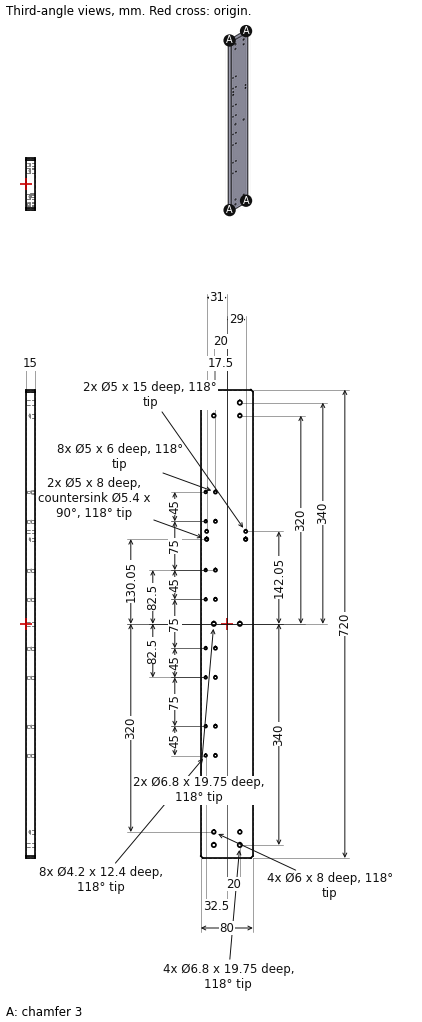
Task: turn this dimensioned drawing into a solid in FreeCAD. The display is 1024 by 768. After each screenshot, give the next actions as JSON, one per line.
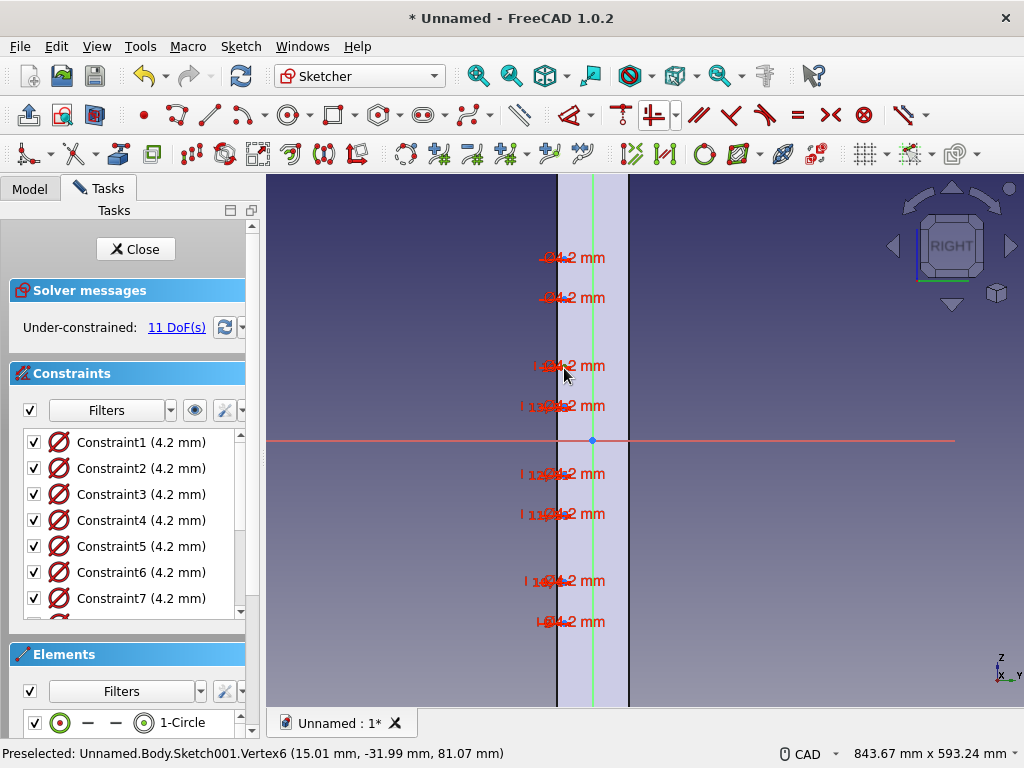
{"action": "left_click", "coordinate": [564, 300]}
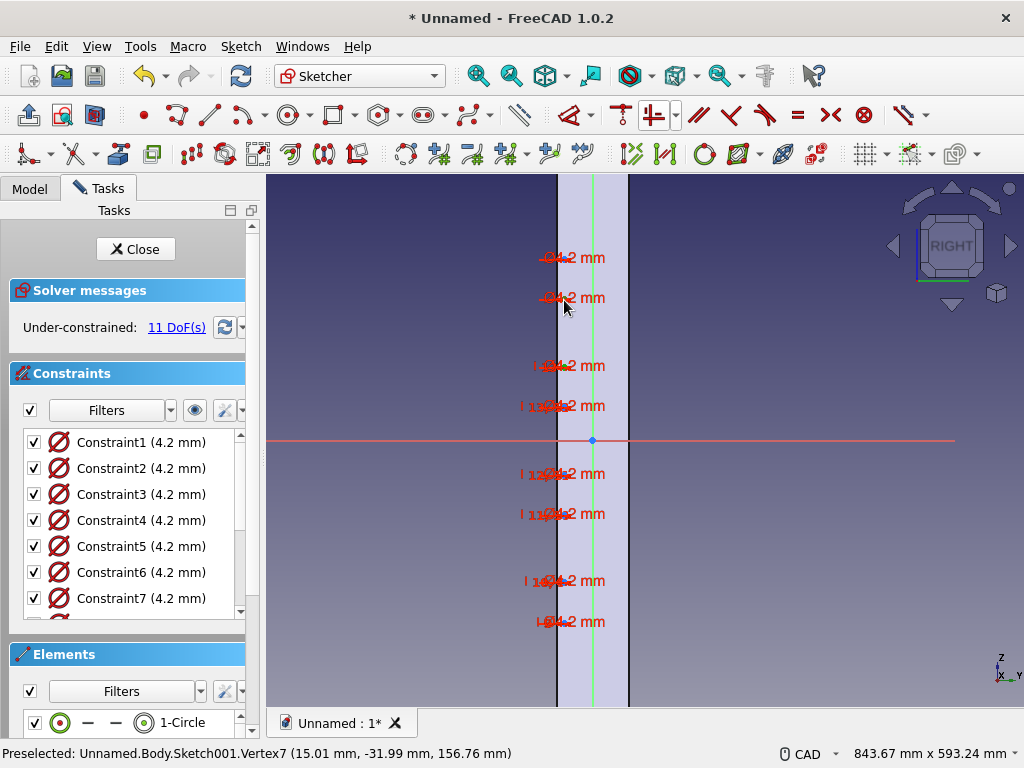
{"action": "left_click", "coordinate": [676, 116]}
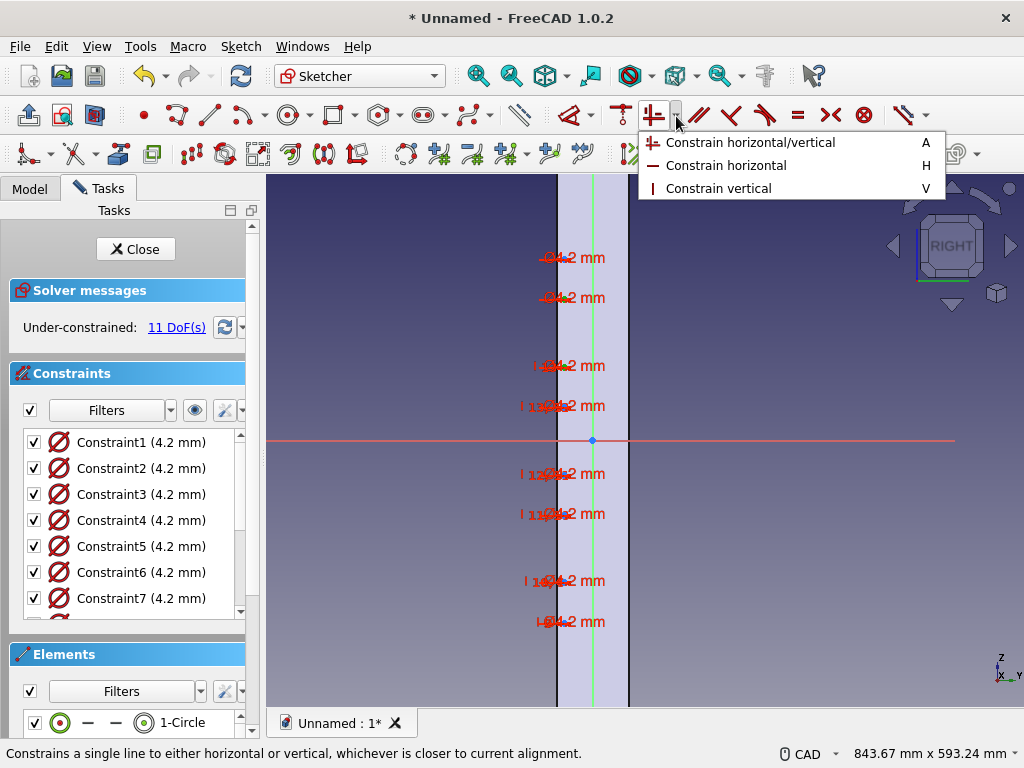
{"action": "left_click", "coordinate": [792, 188]}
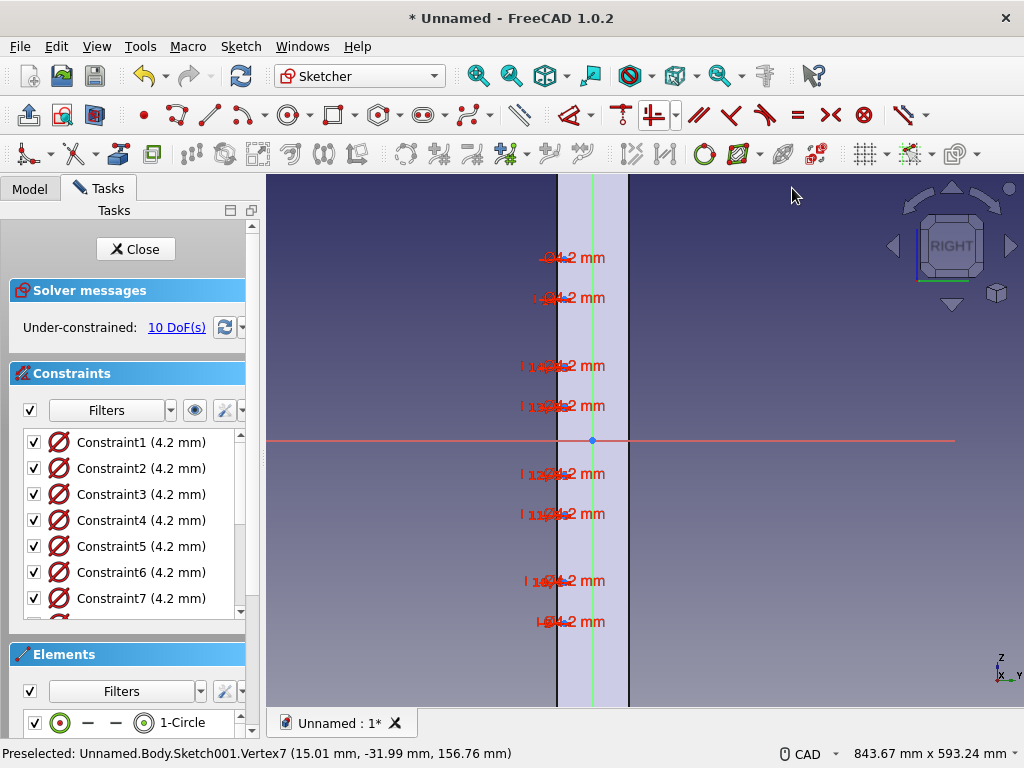
{"action": "left_click", "coordinate": [564, 300]}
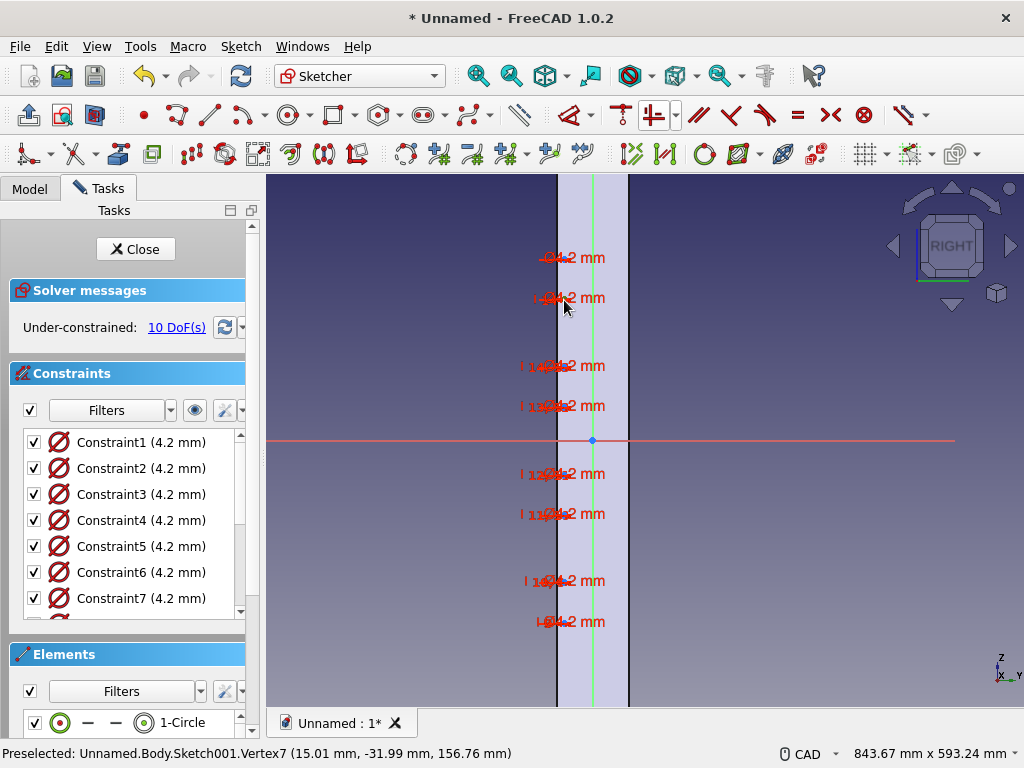
{"action": "left_click", "coordinate": [564, 260]}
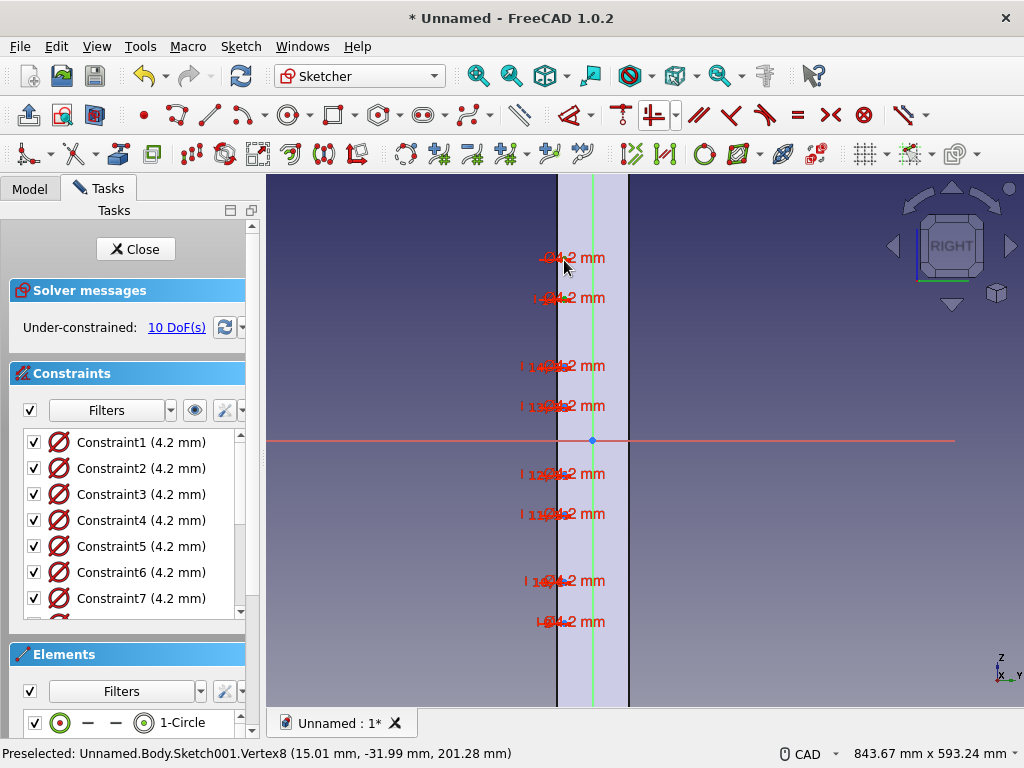
{"action": "key", "text": "v"}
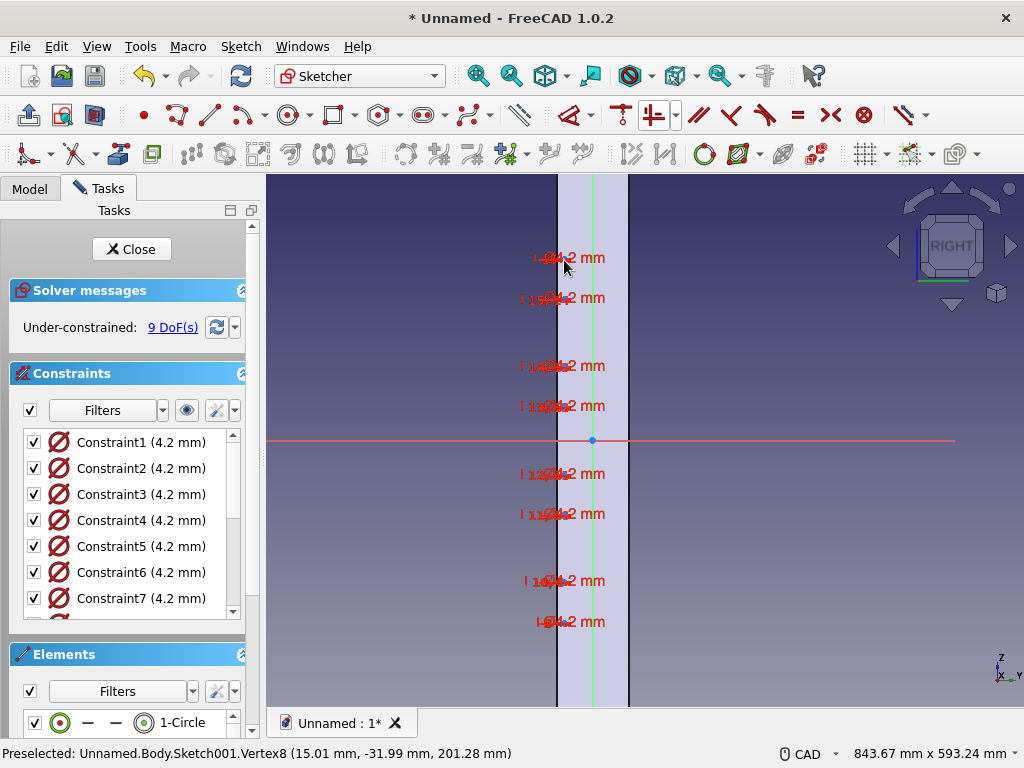
{"action": "left_click", "coordinate": [564, 624]}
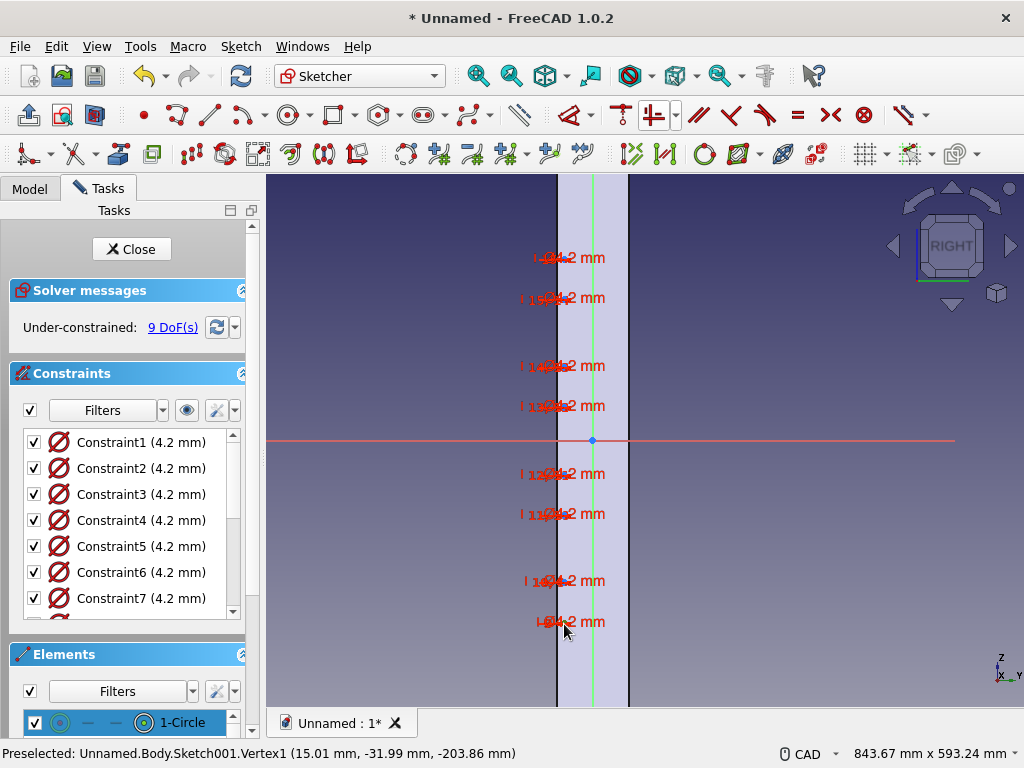
{"action": "left_click", "coordinate": [564, 583]}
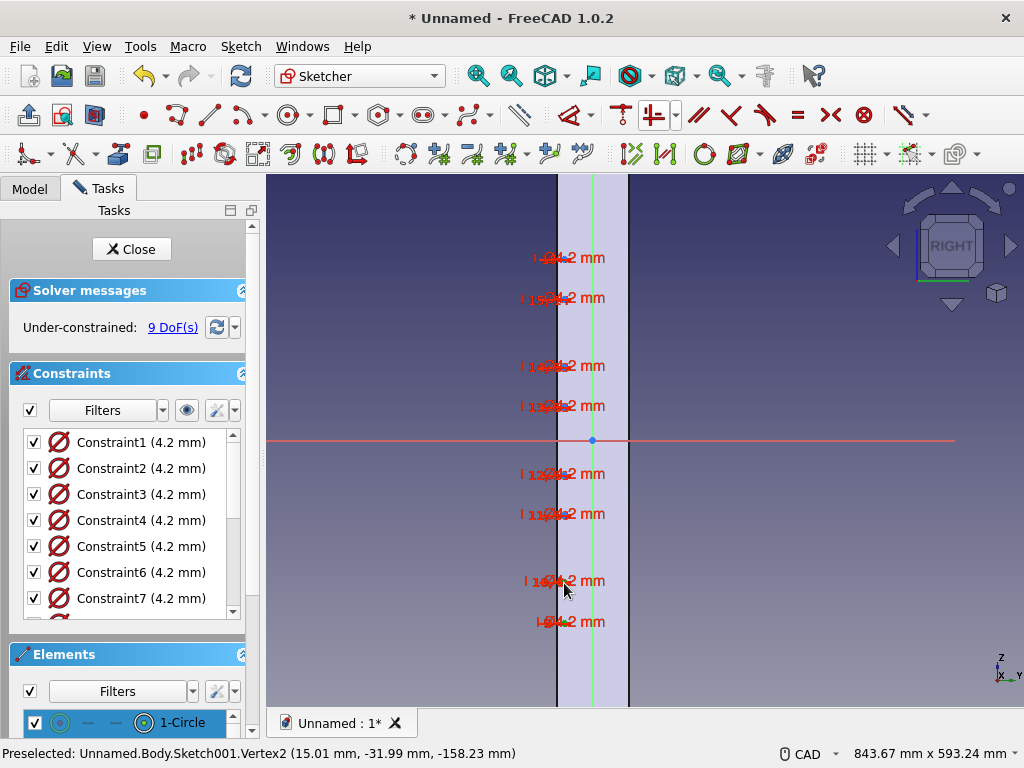
{"action": "key", "text": "i"}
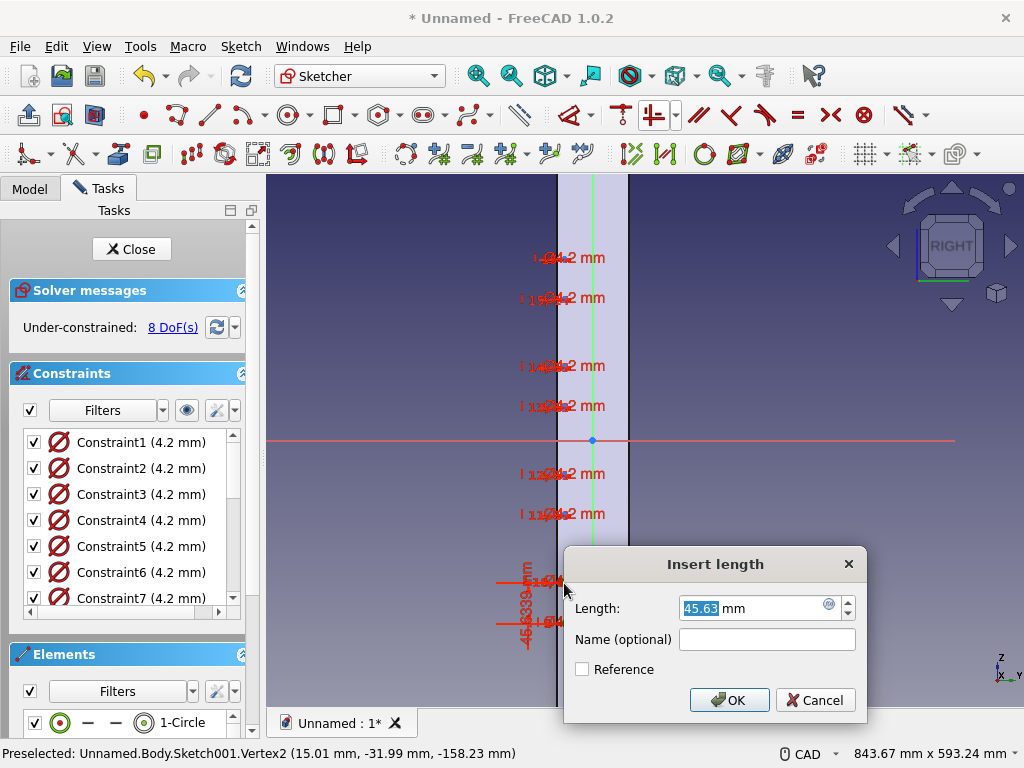
{"action": "type", "text": "45"}
{"action": "key", "text": "Return"}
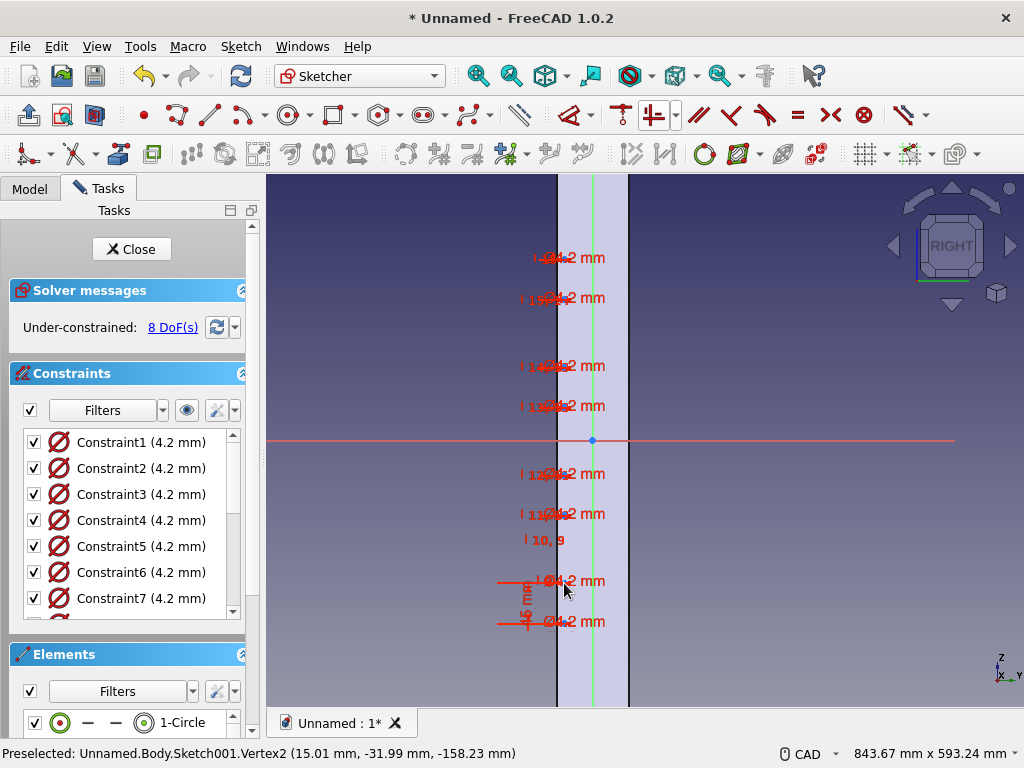
{"action": "left_click", "coordinate": [564, 583]}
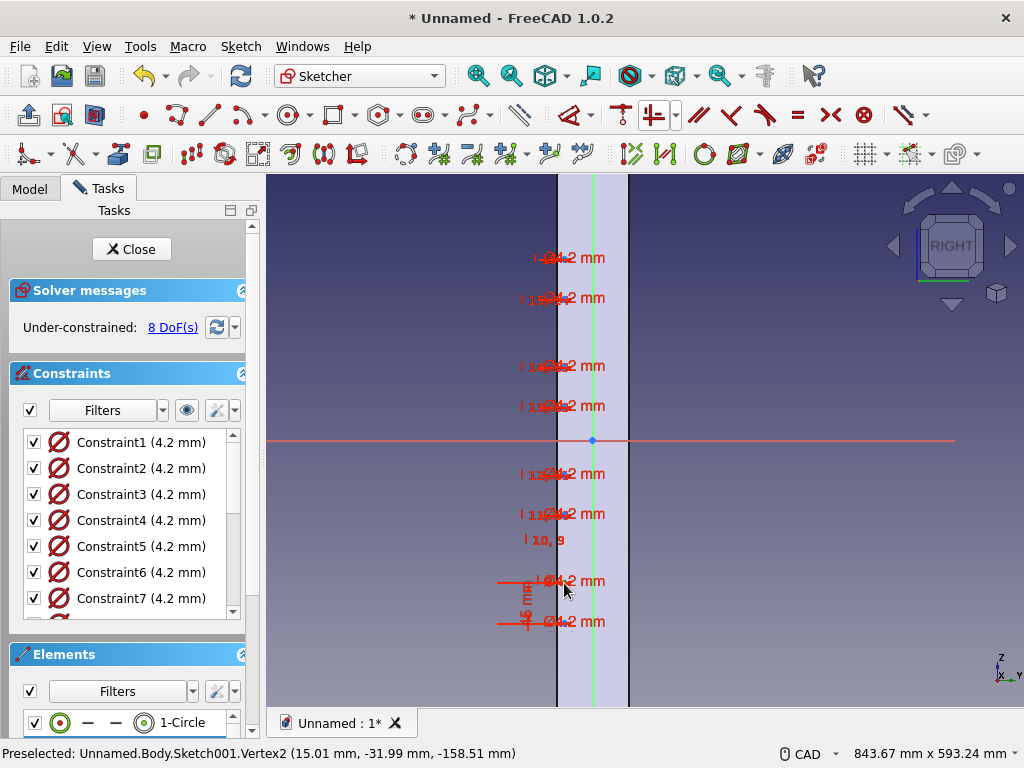
{"action": "left_click", "coordinate": [564, 516]}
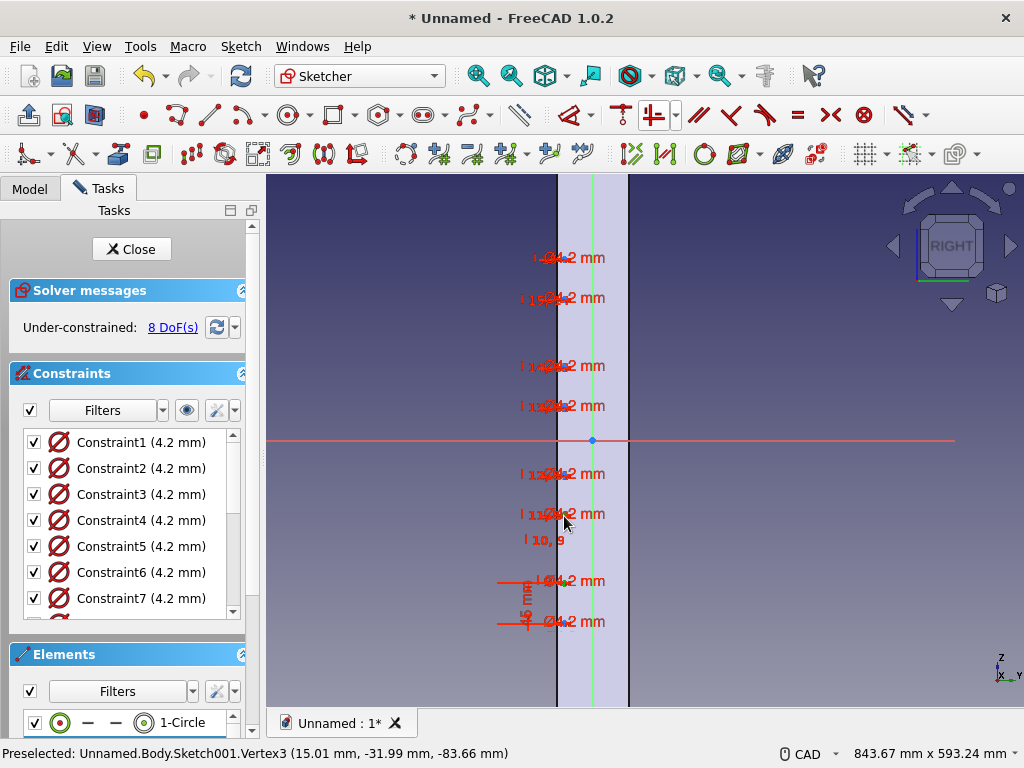
{"action": "key", "text": "i"}